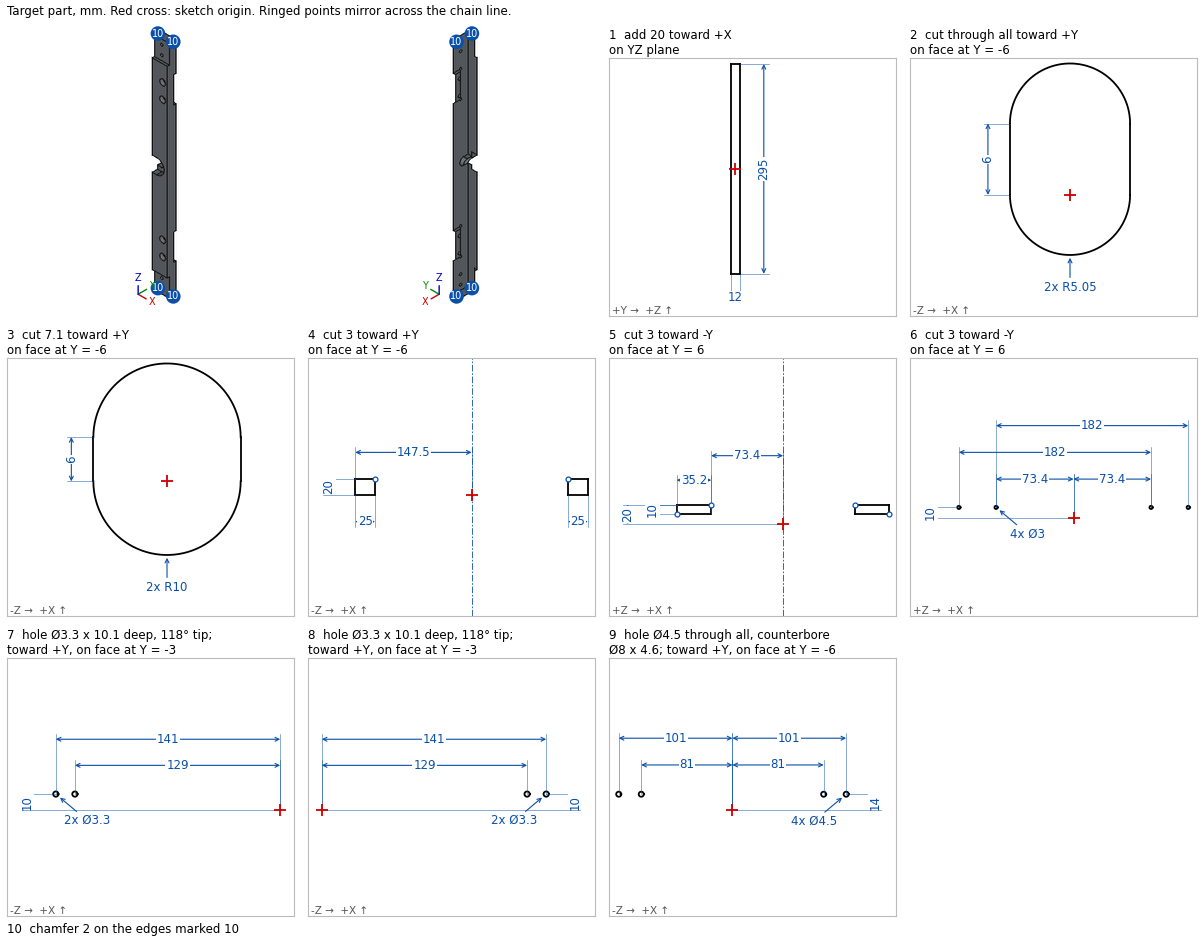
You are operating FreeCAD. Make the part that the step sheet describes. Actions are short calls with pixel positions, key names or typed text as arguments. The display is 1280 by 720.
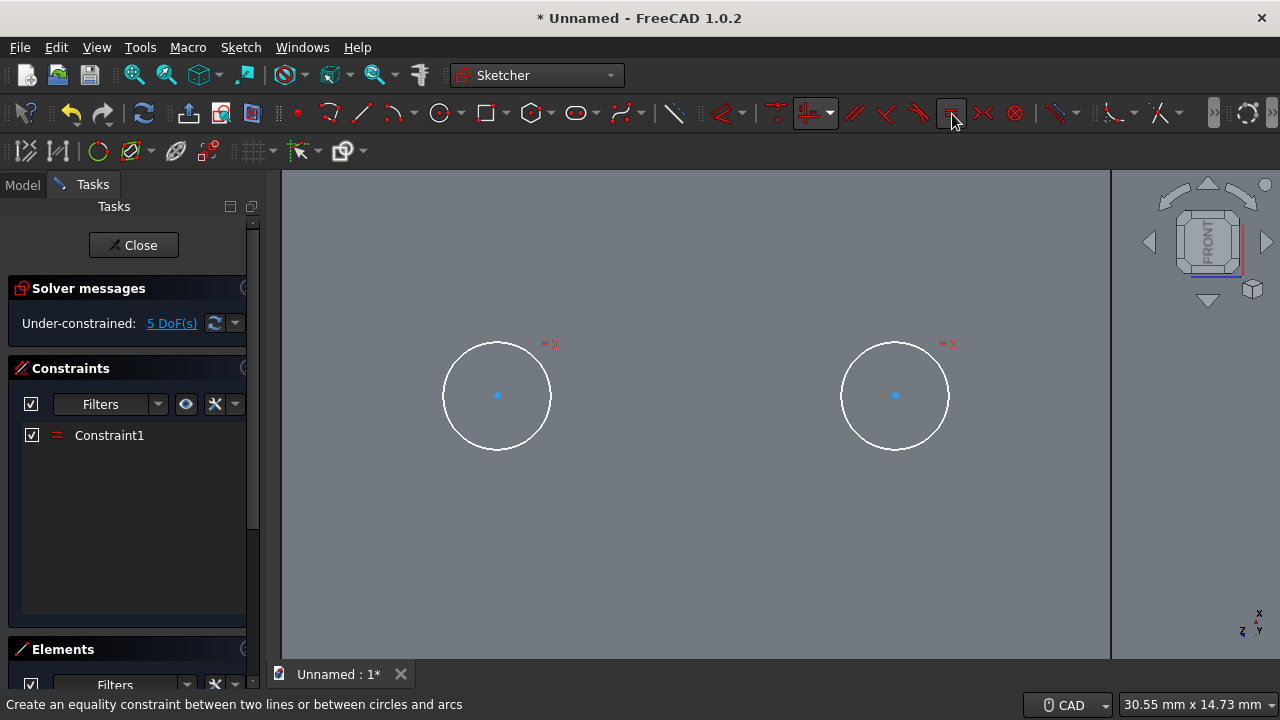
click(497, 396)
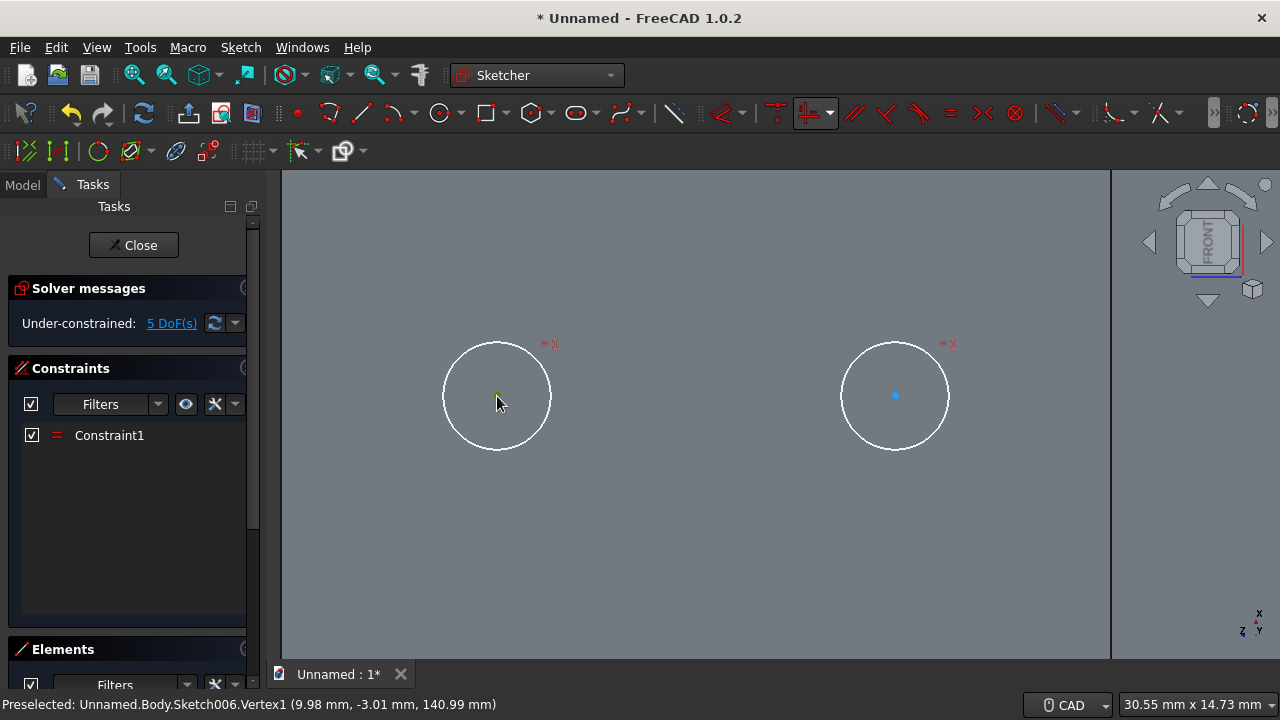
click(895, 396)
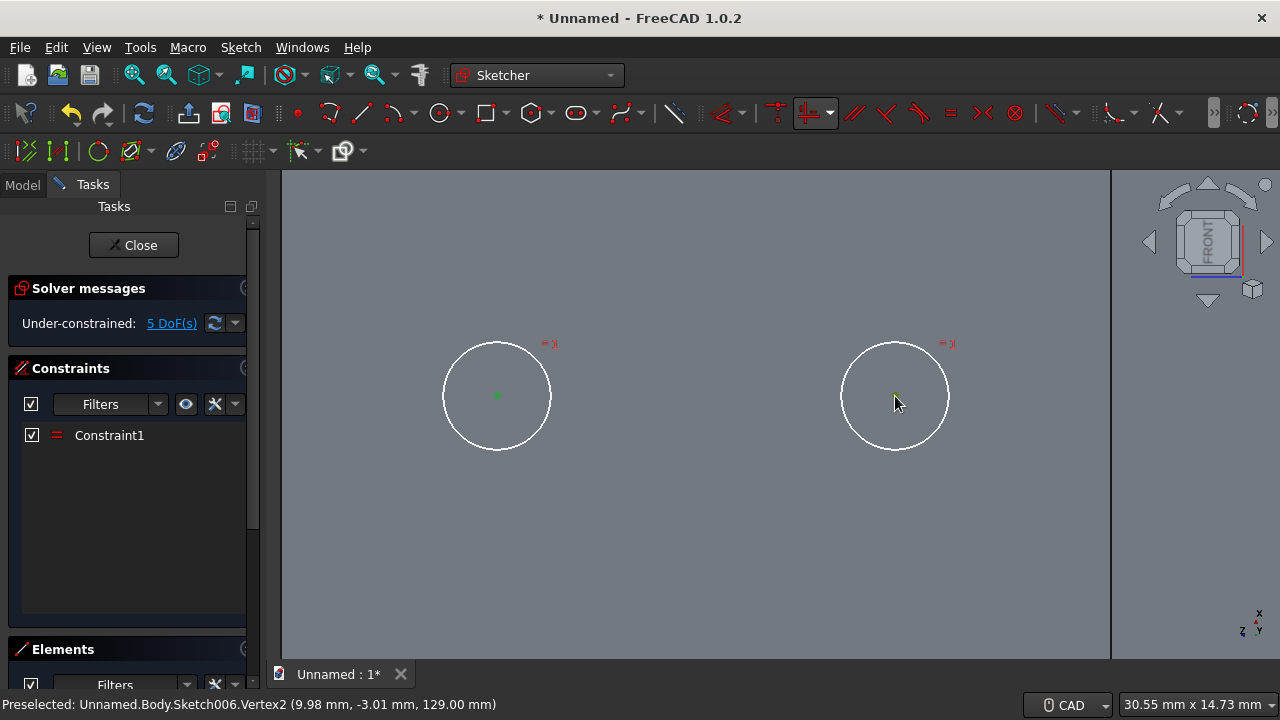
key(h)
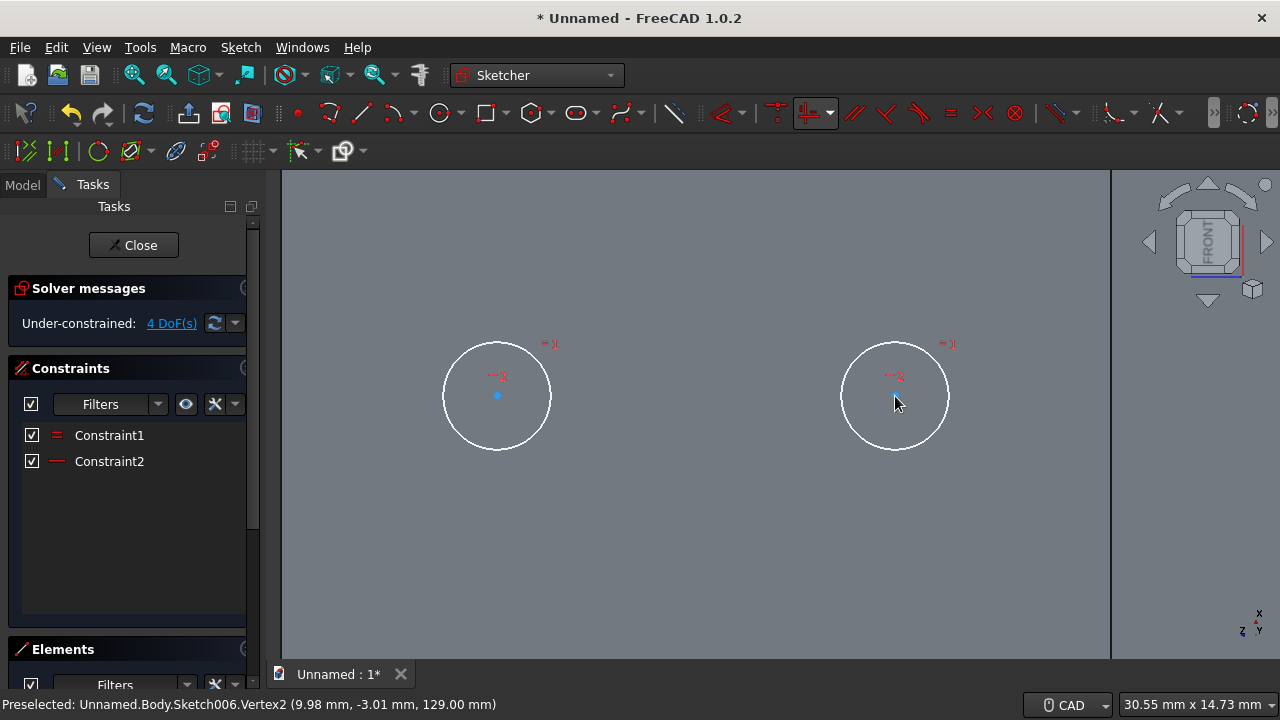
click(722, 114)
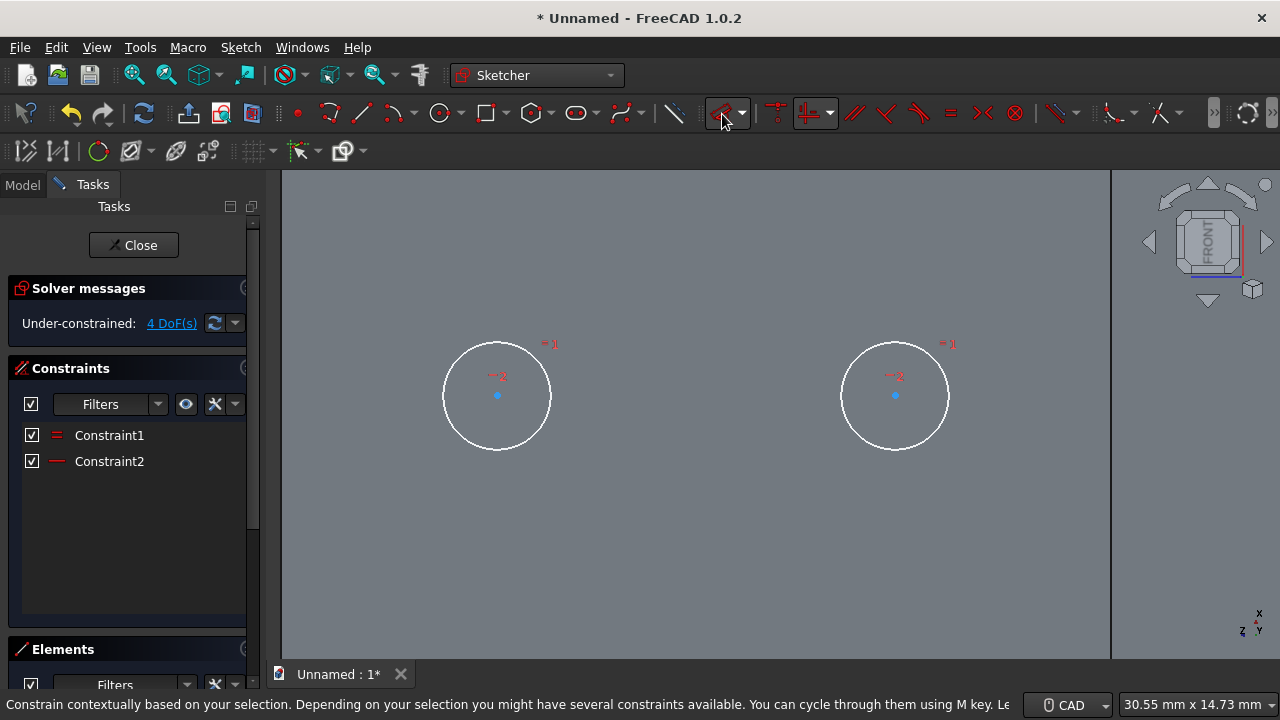
click(535, 358)
click(558, 335)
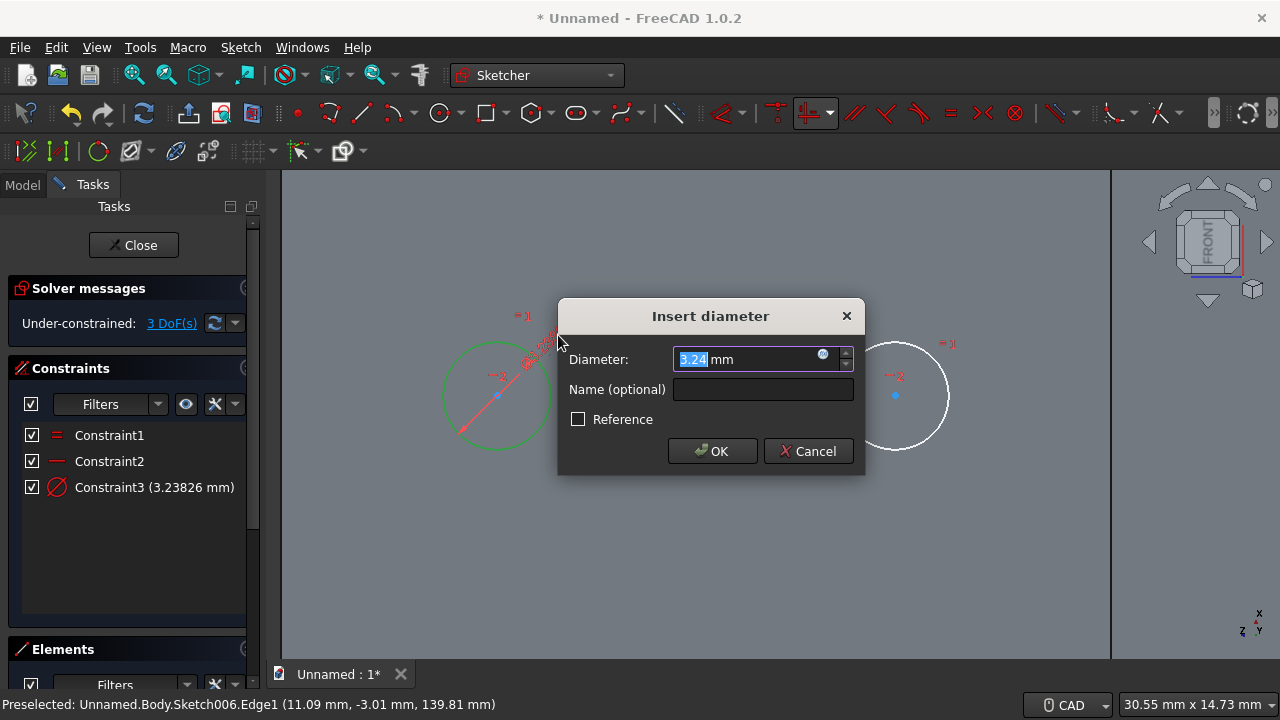
text(3.3)
key(Return)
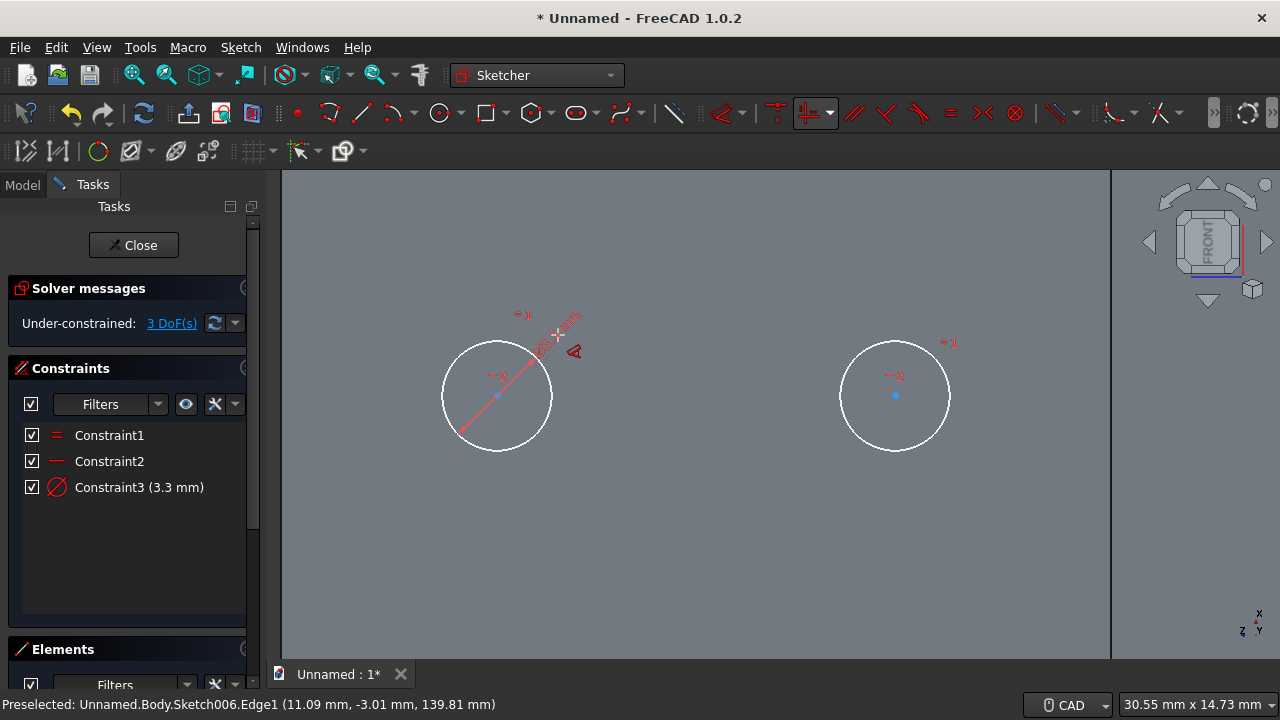
click(497, 396)
click(463, 514)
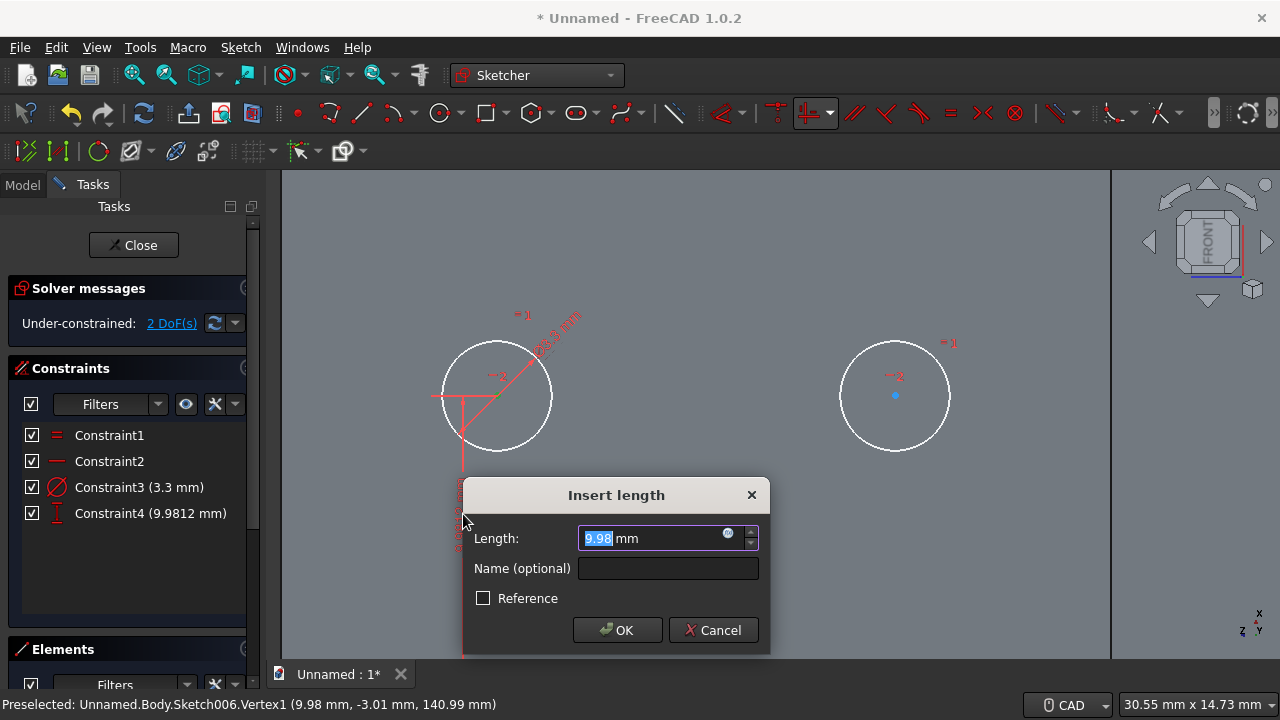
text(10)
key(Return)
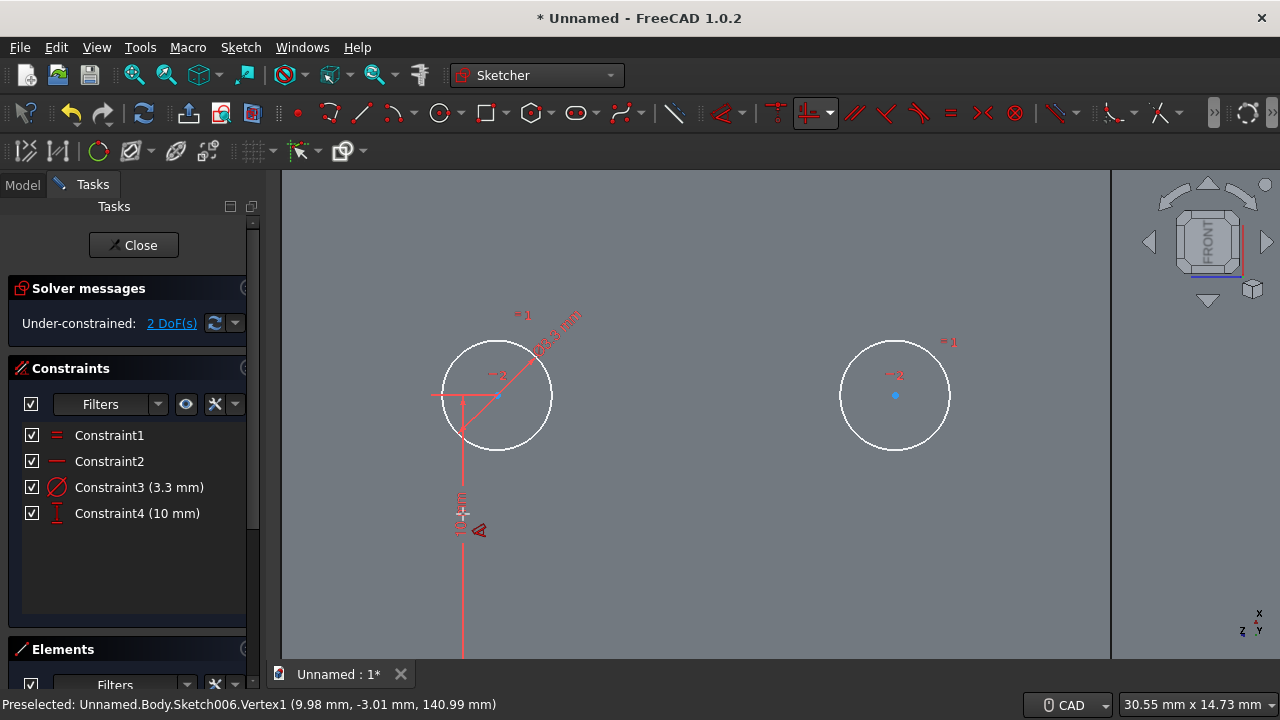
click(497, 395)
click(806, 361)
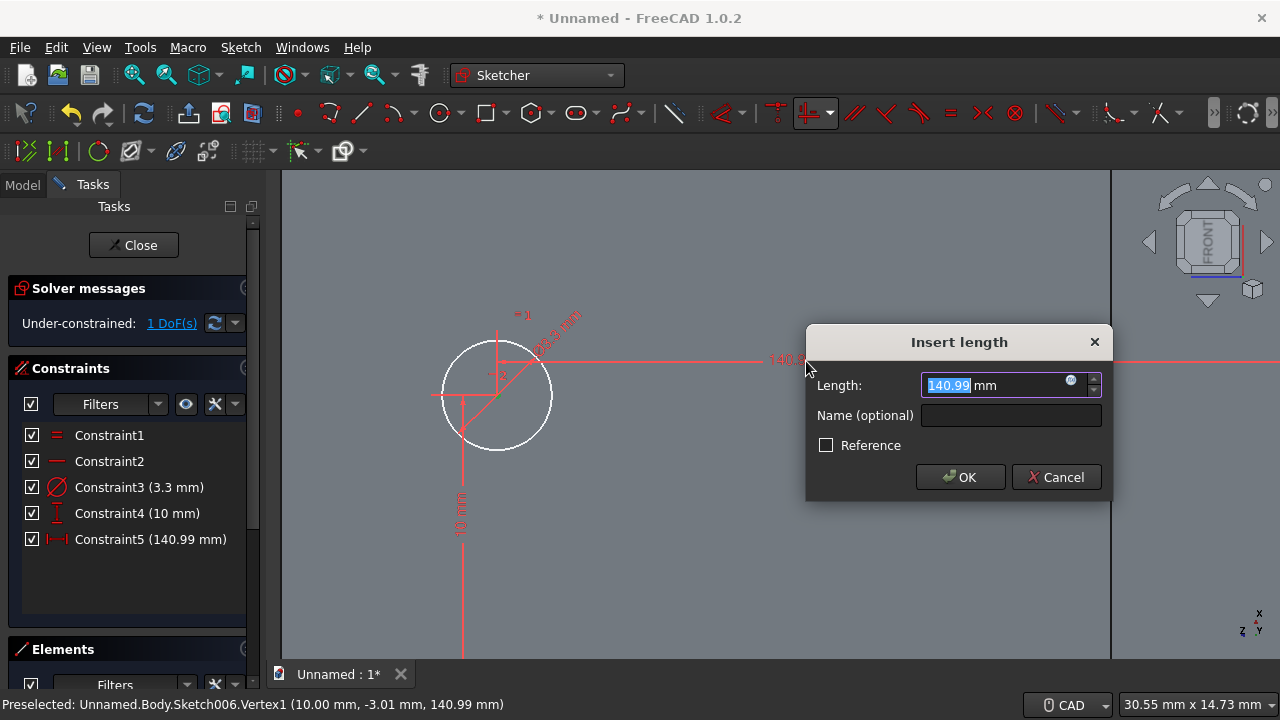
text(141)
key(Return)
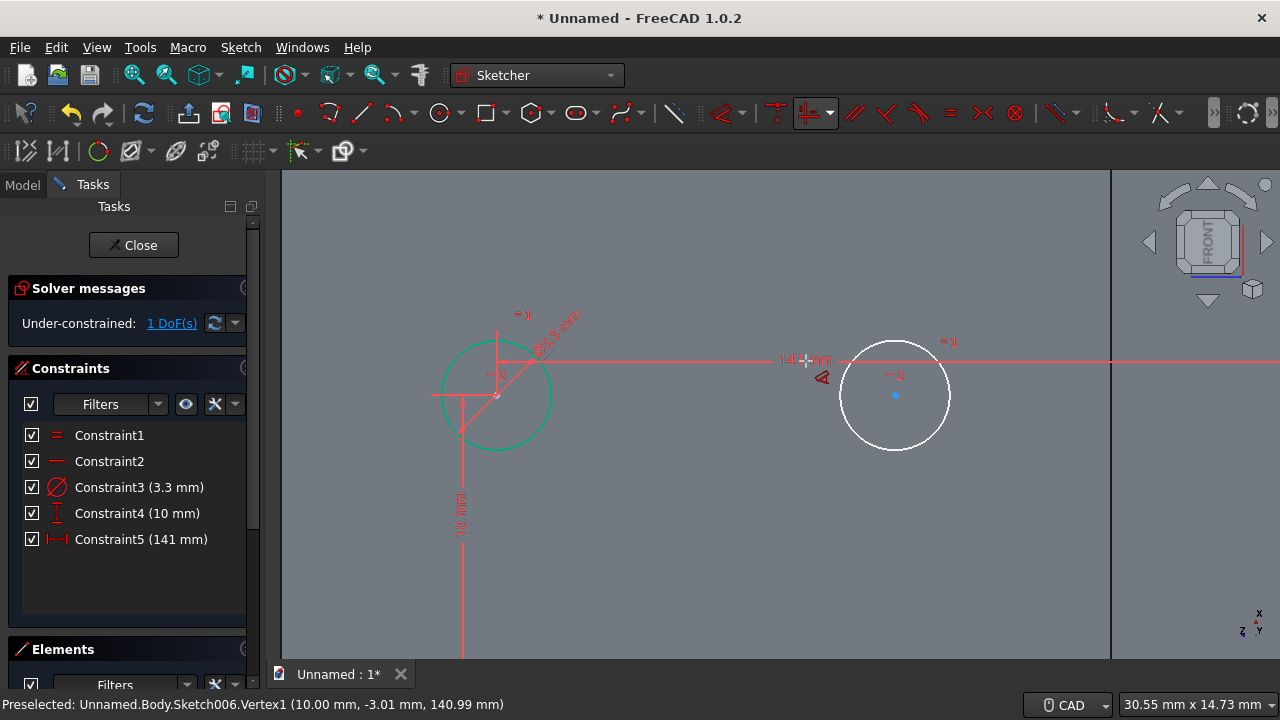
click(895, 395)
click(1005, 361)